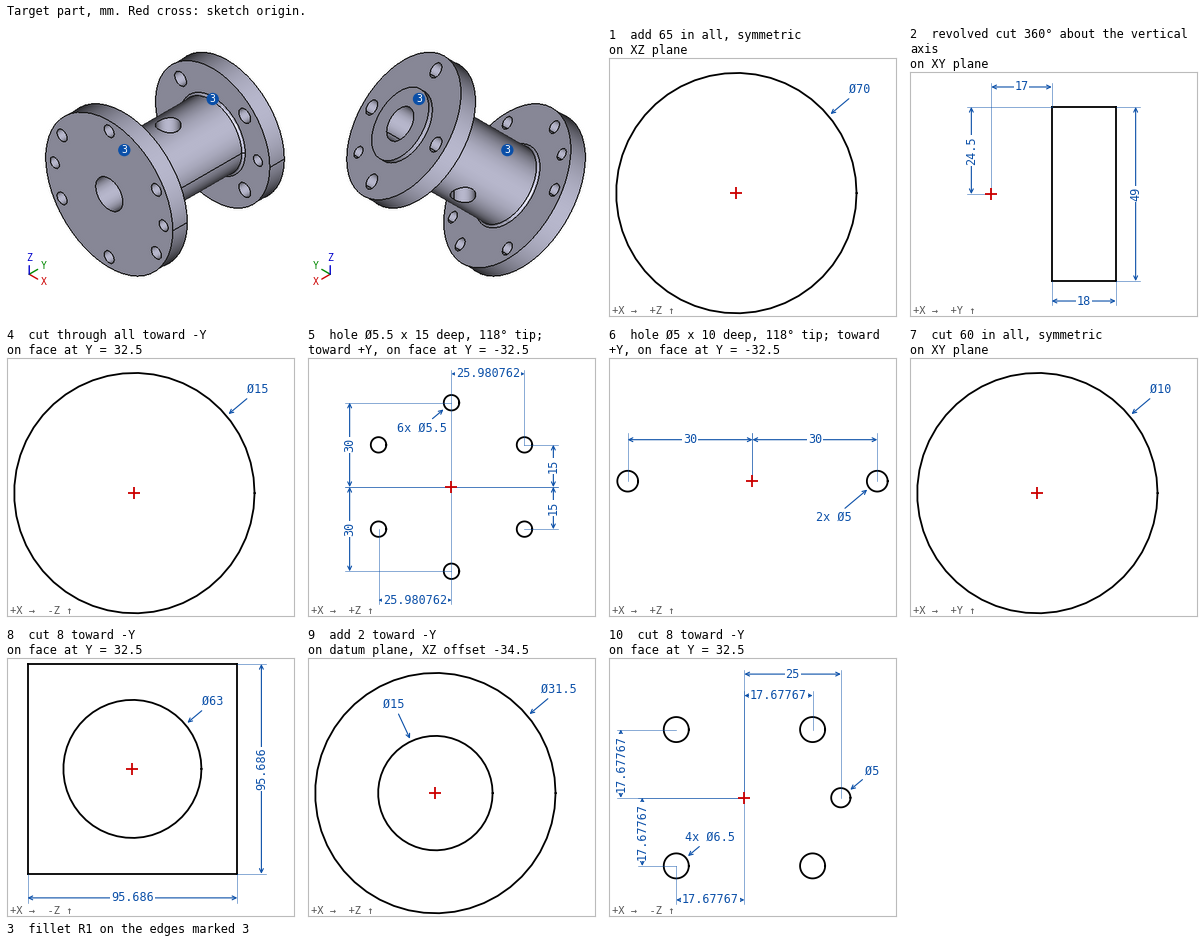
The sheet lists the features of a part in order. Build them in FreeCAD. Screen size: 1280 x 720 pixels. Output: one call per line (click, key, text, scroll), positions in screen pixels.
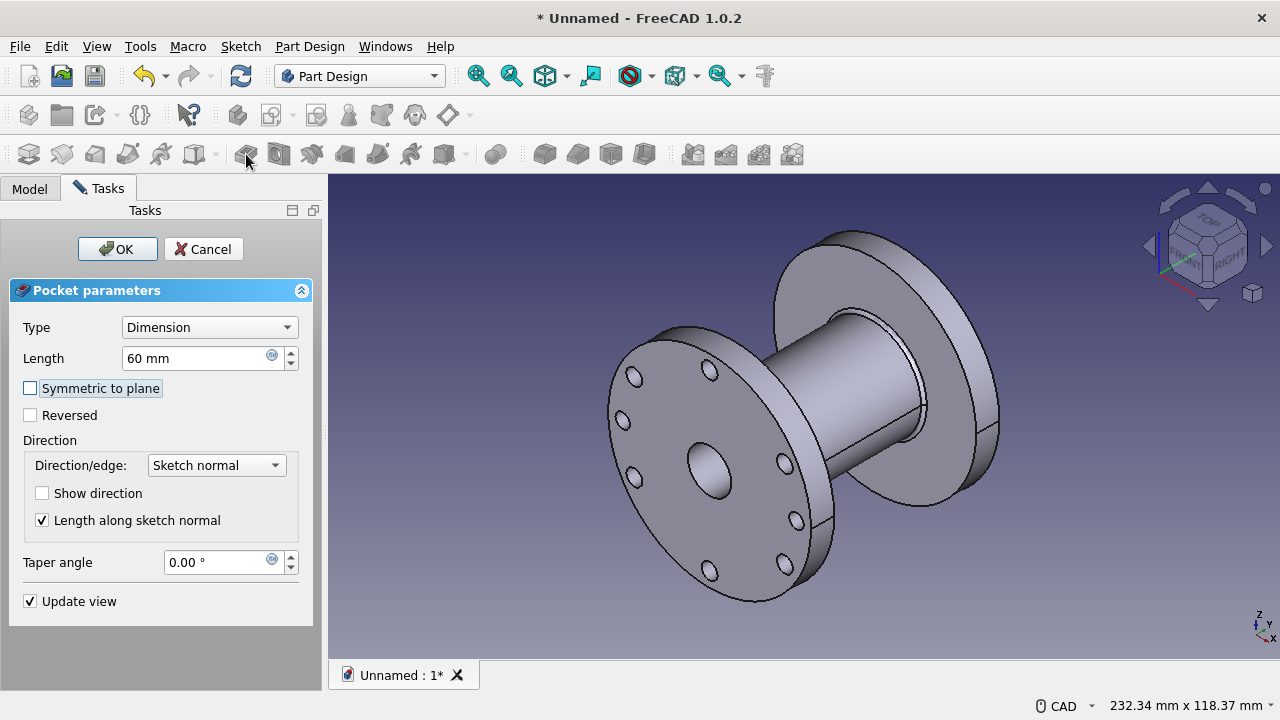
click(31, 388)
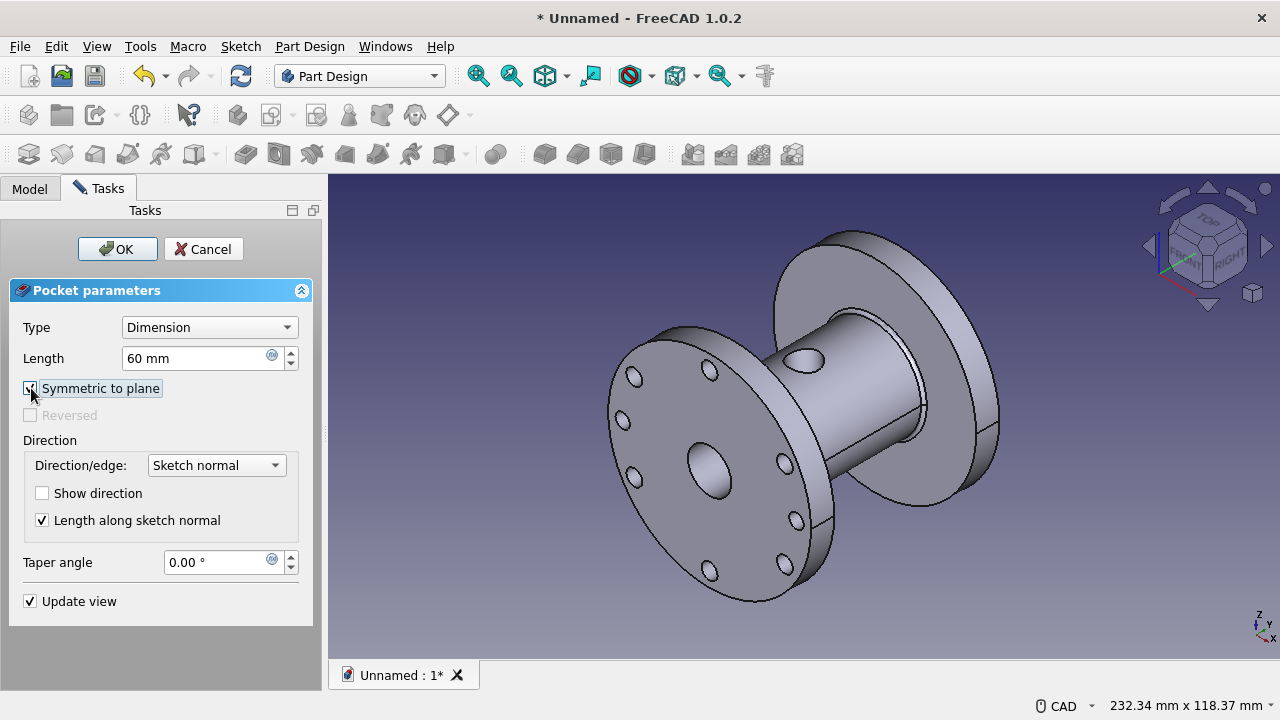
click(118, 249)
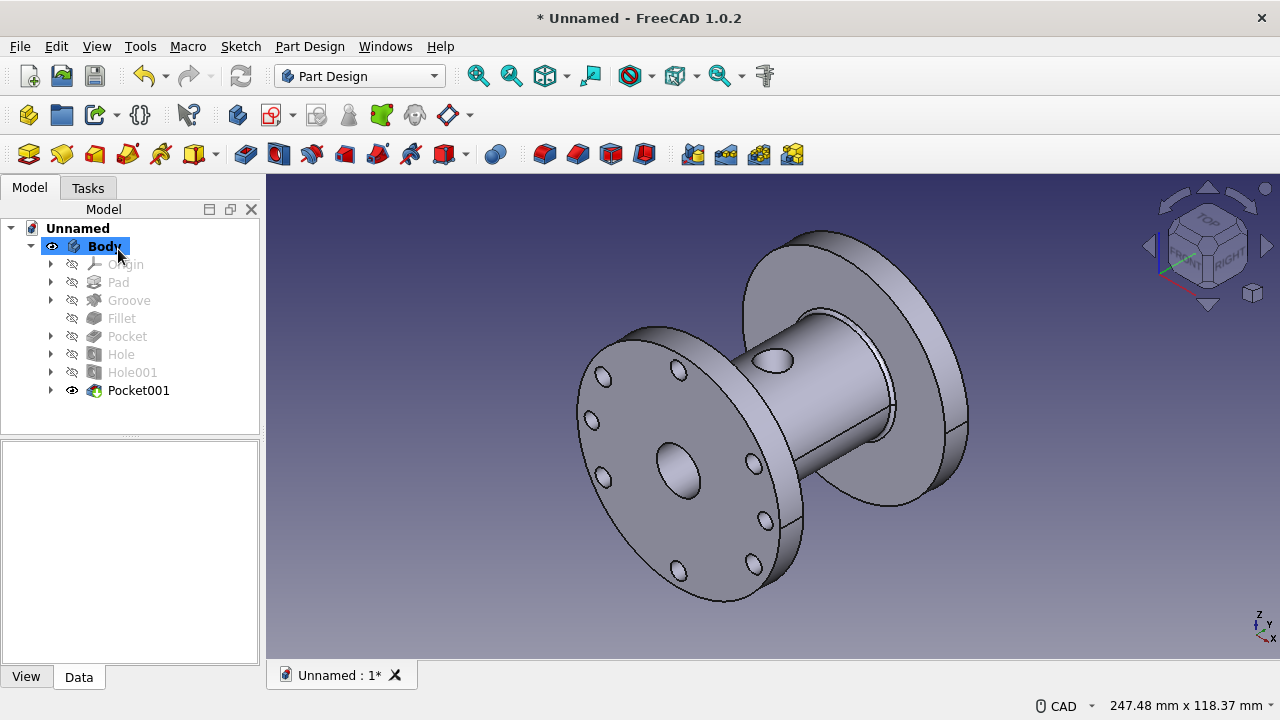
key(4)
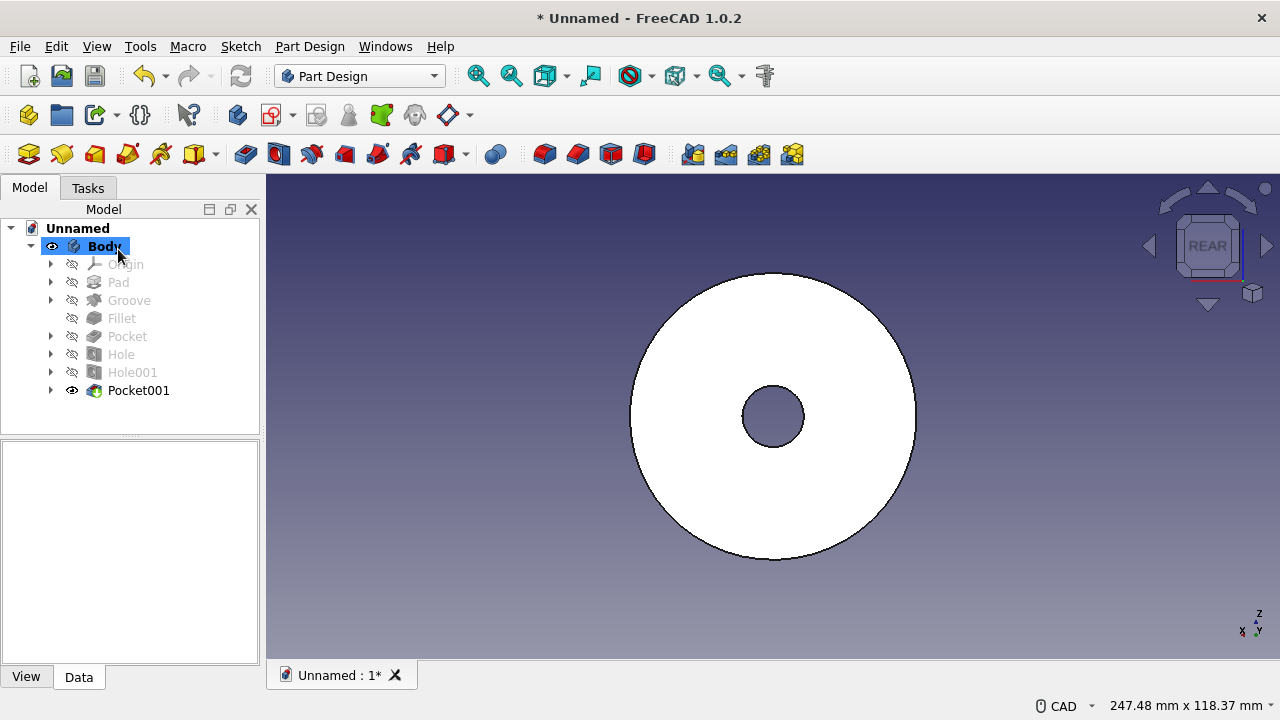
click(732, 497)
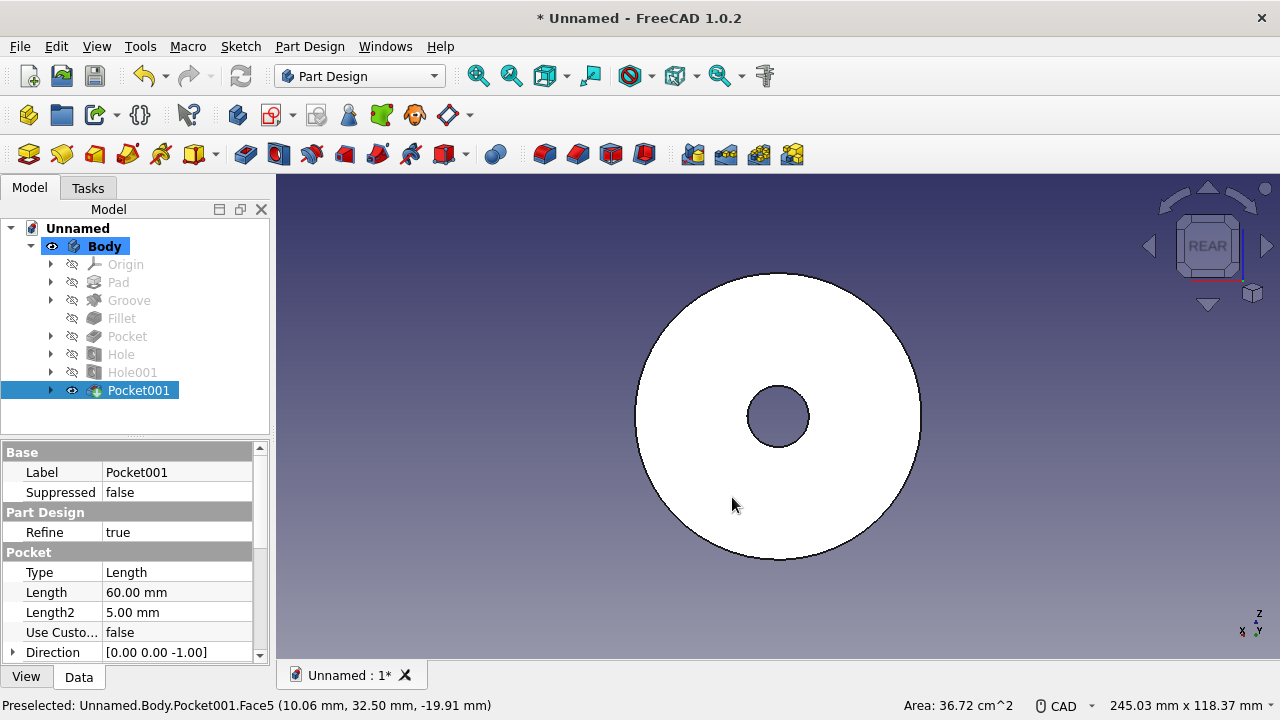
click(270, 116)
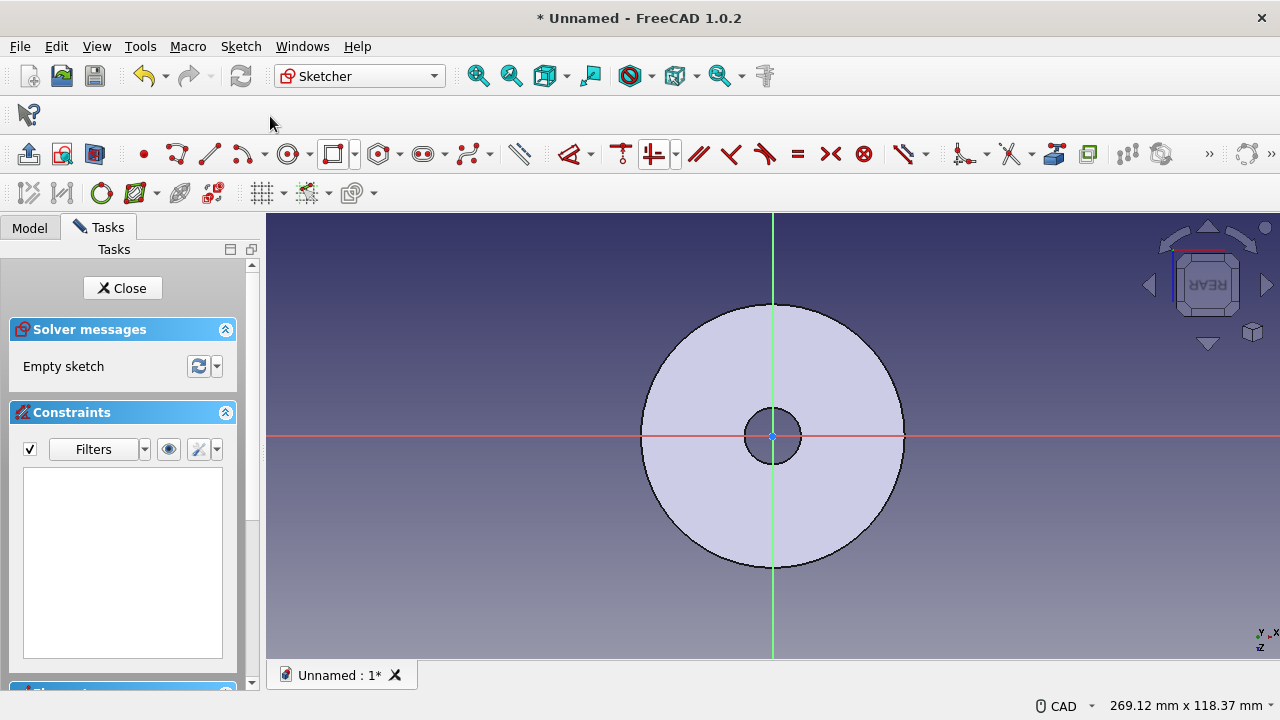
scroll(396, 436, down, 1)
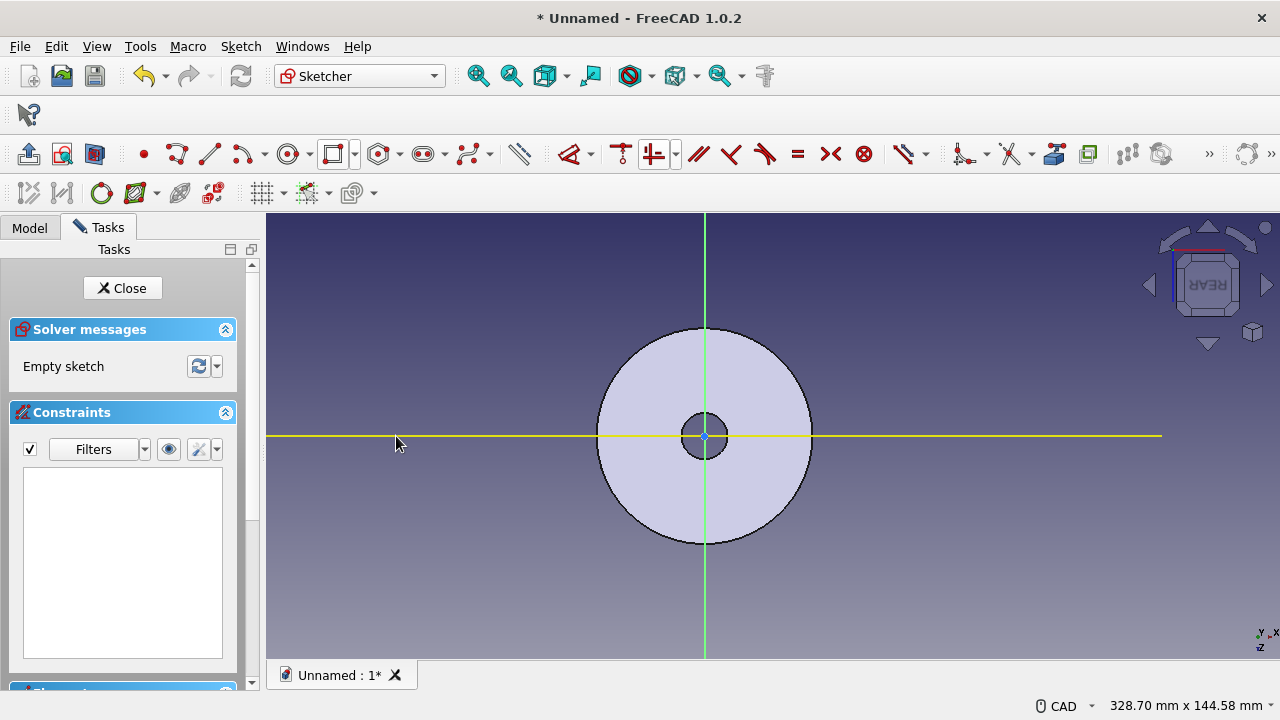
key(g)
key(v)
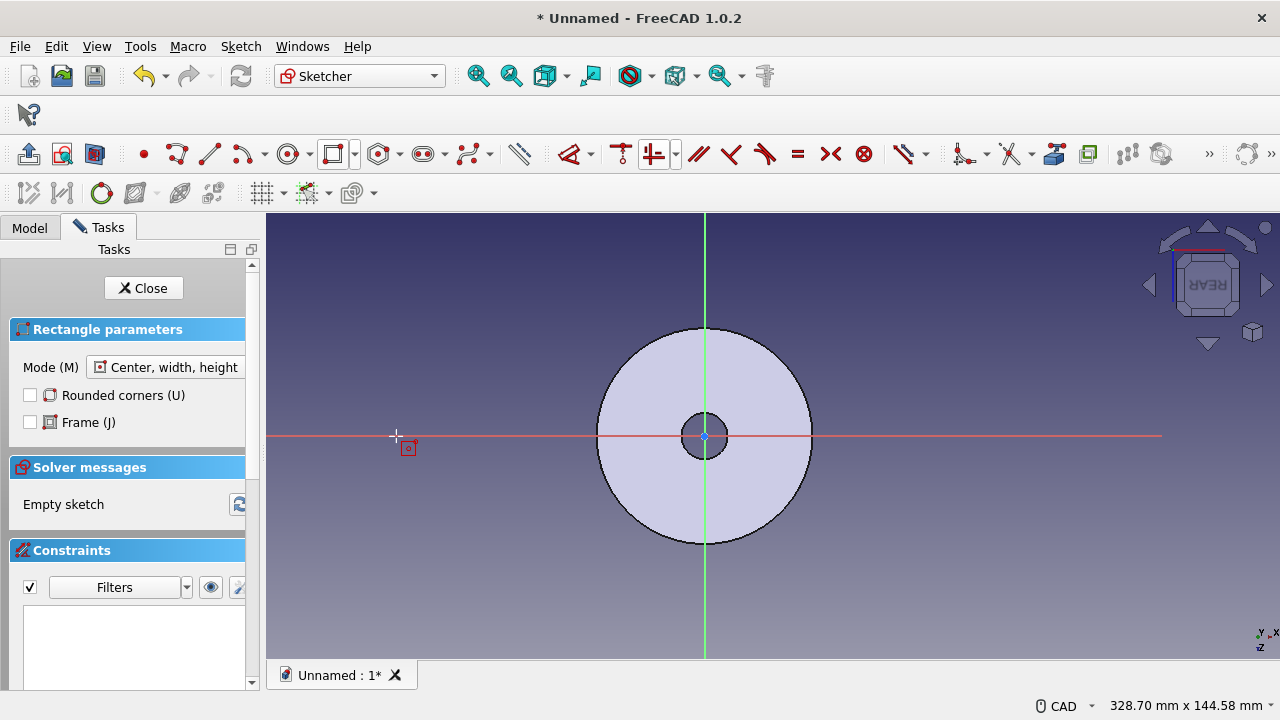
click(705, 436)
move(852, 289)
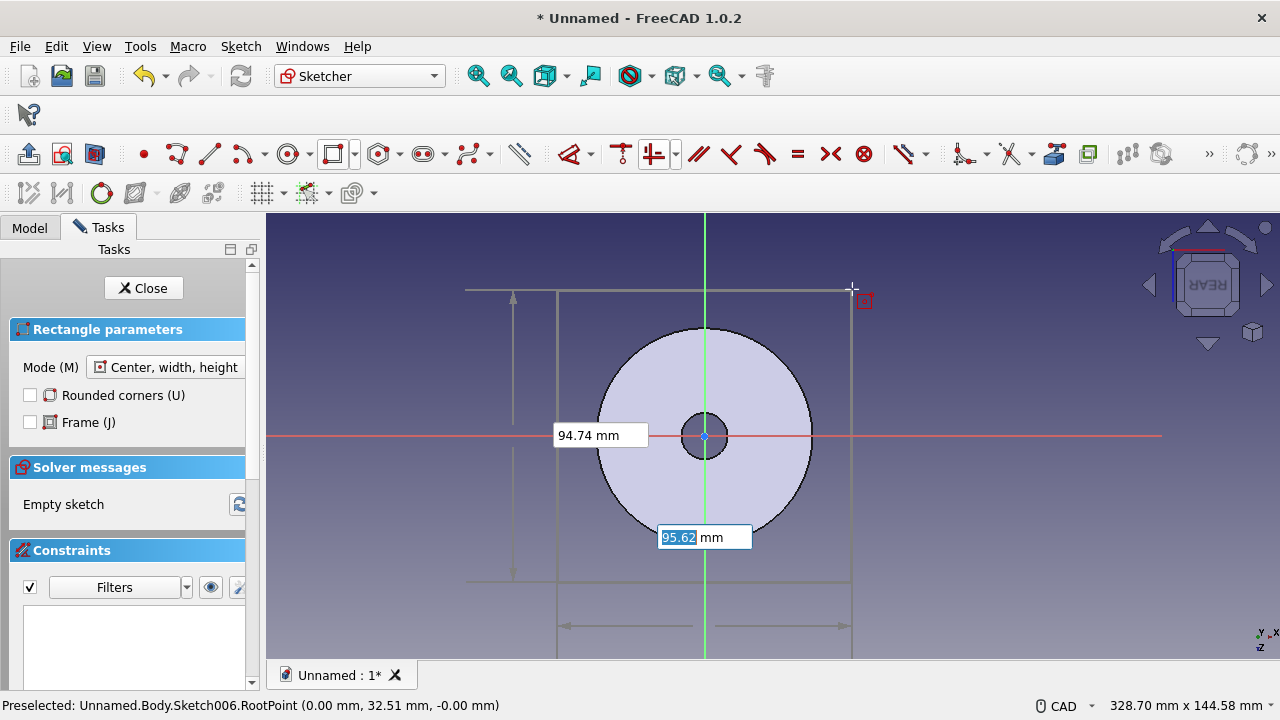
text(95.686)
key(Tab)
text(95.686)
key(Return)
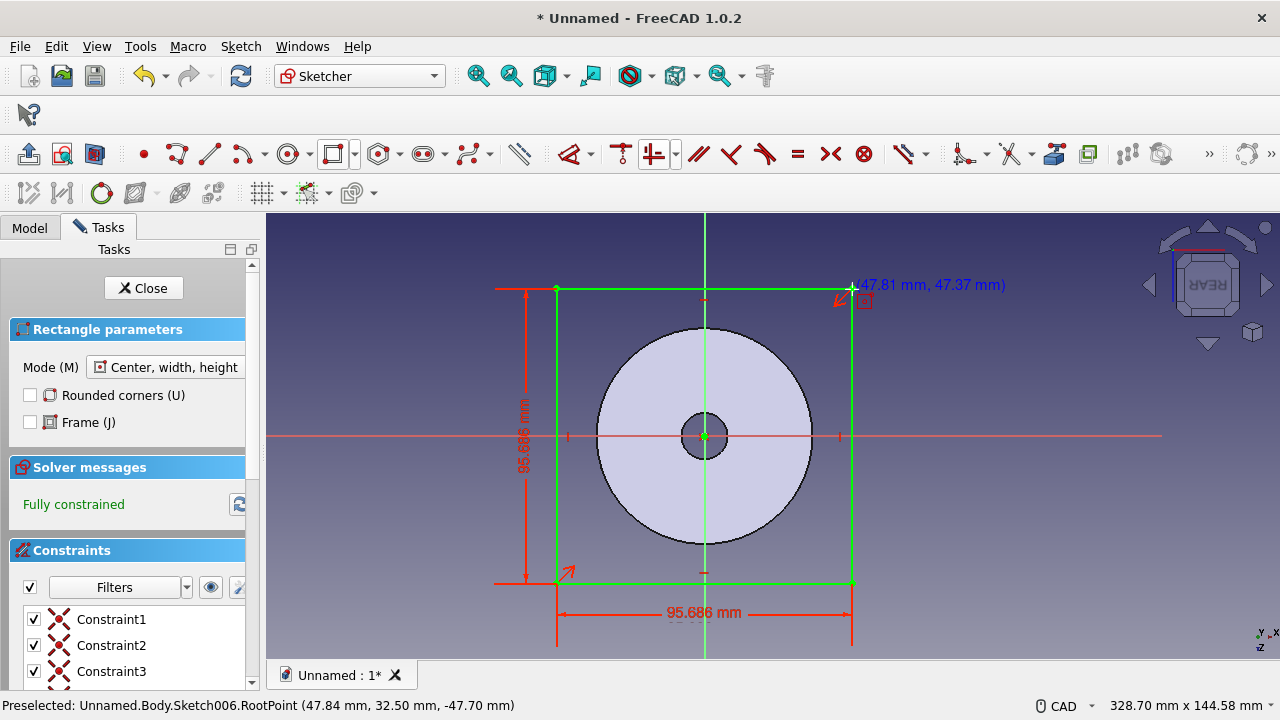
click(288, 154)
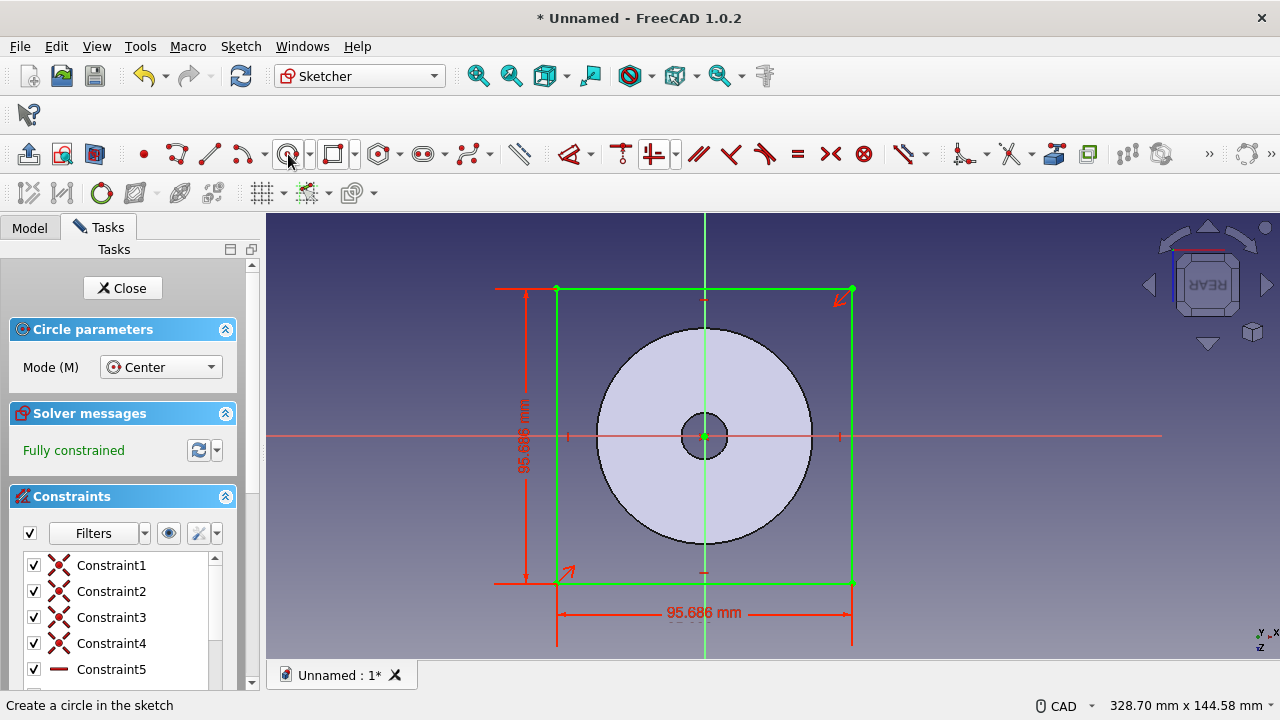
click(705, 436)
move(773, 367)